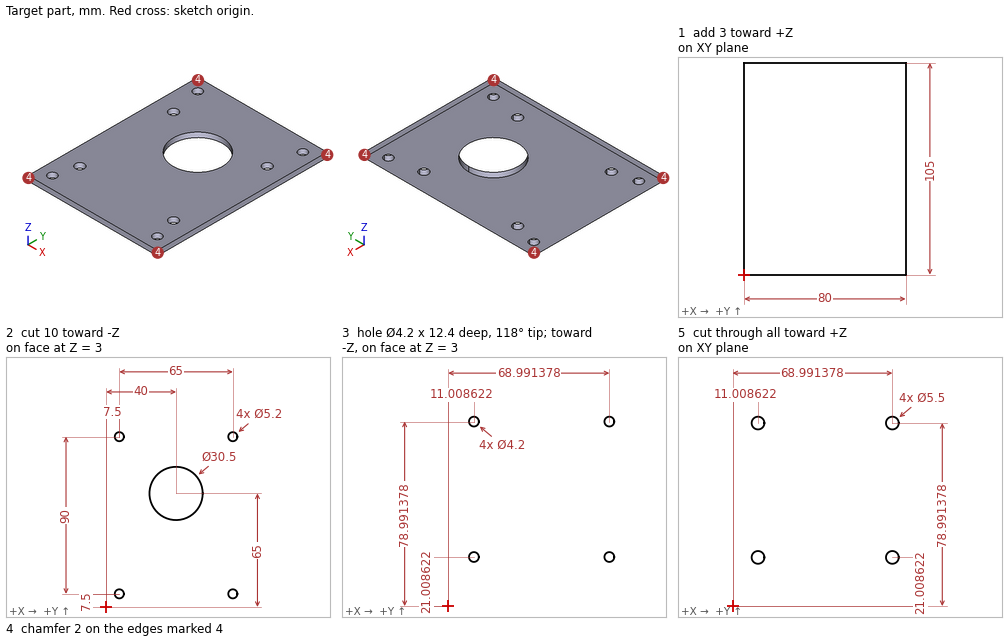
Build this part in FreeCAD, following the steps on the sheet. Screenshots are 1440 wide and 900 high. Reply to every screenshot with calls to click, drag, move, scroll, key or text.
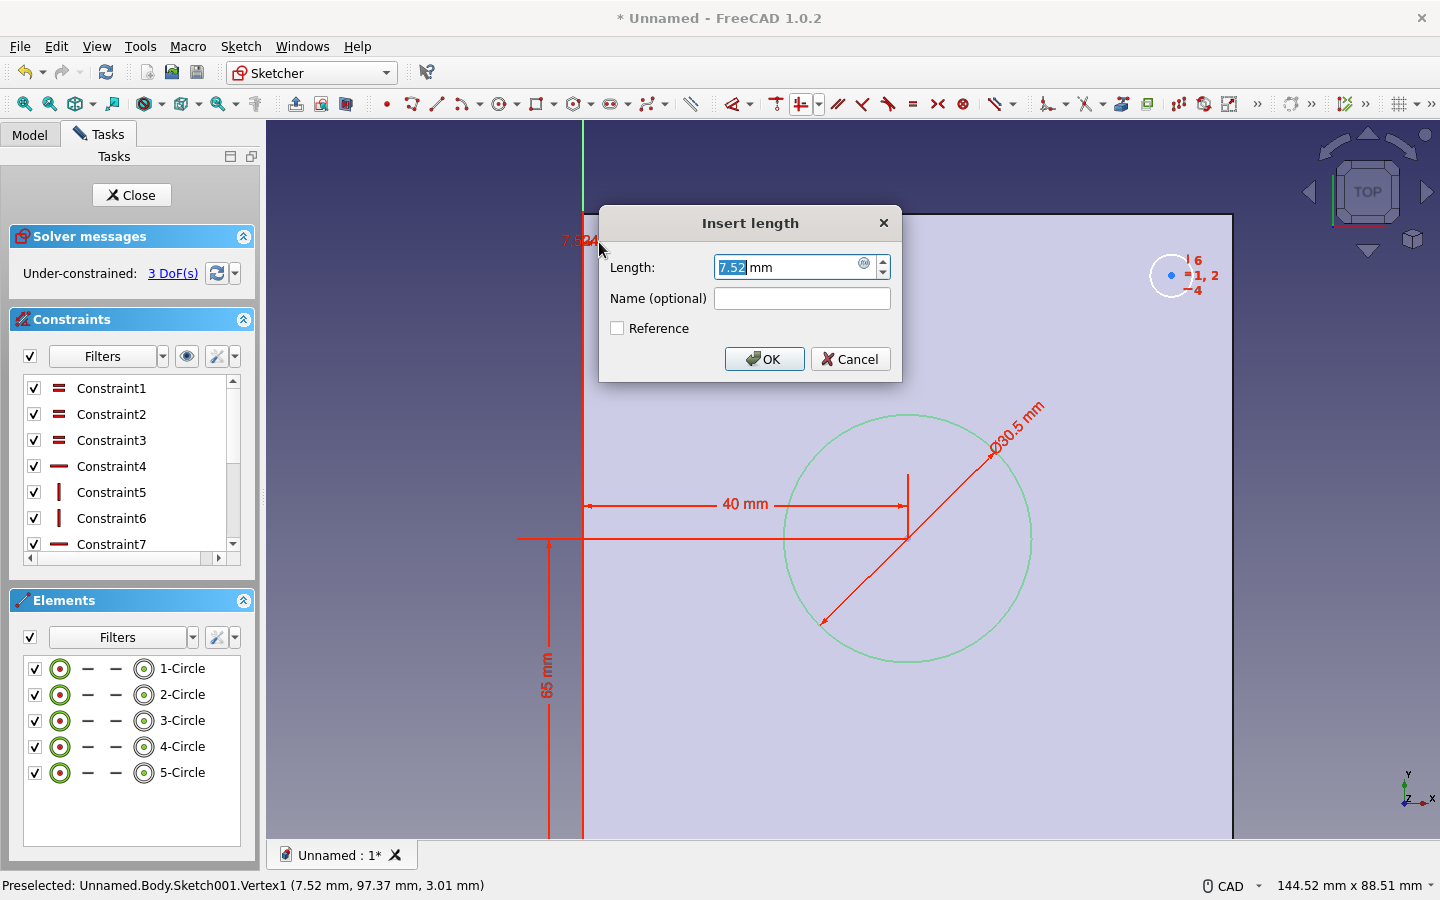
text(7.5)
key(Return)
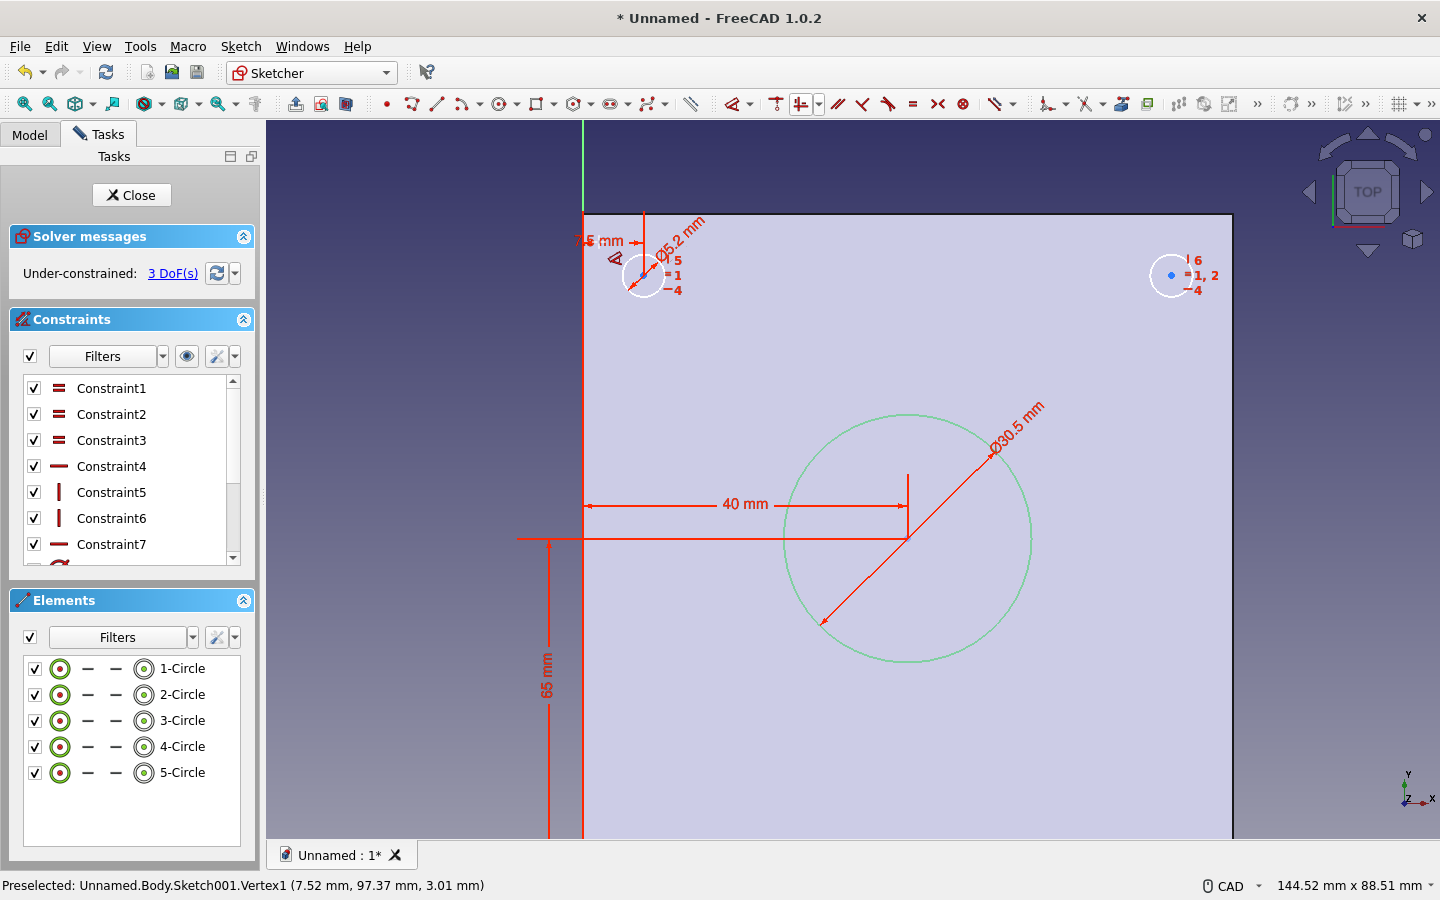
scroll(659, 260, down, 3)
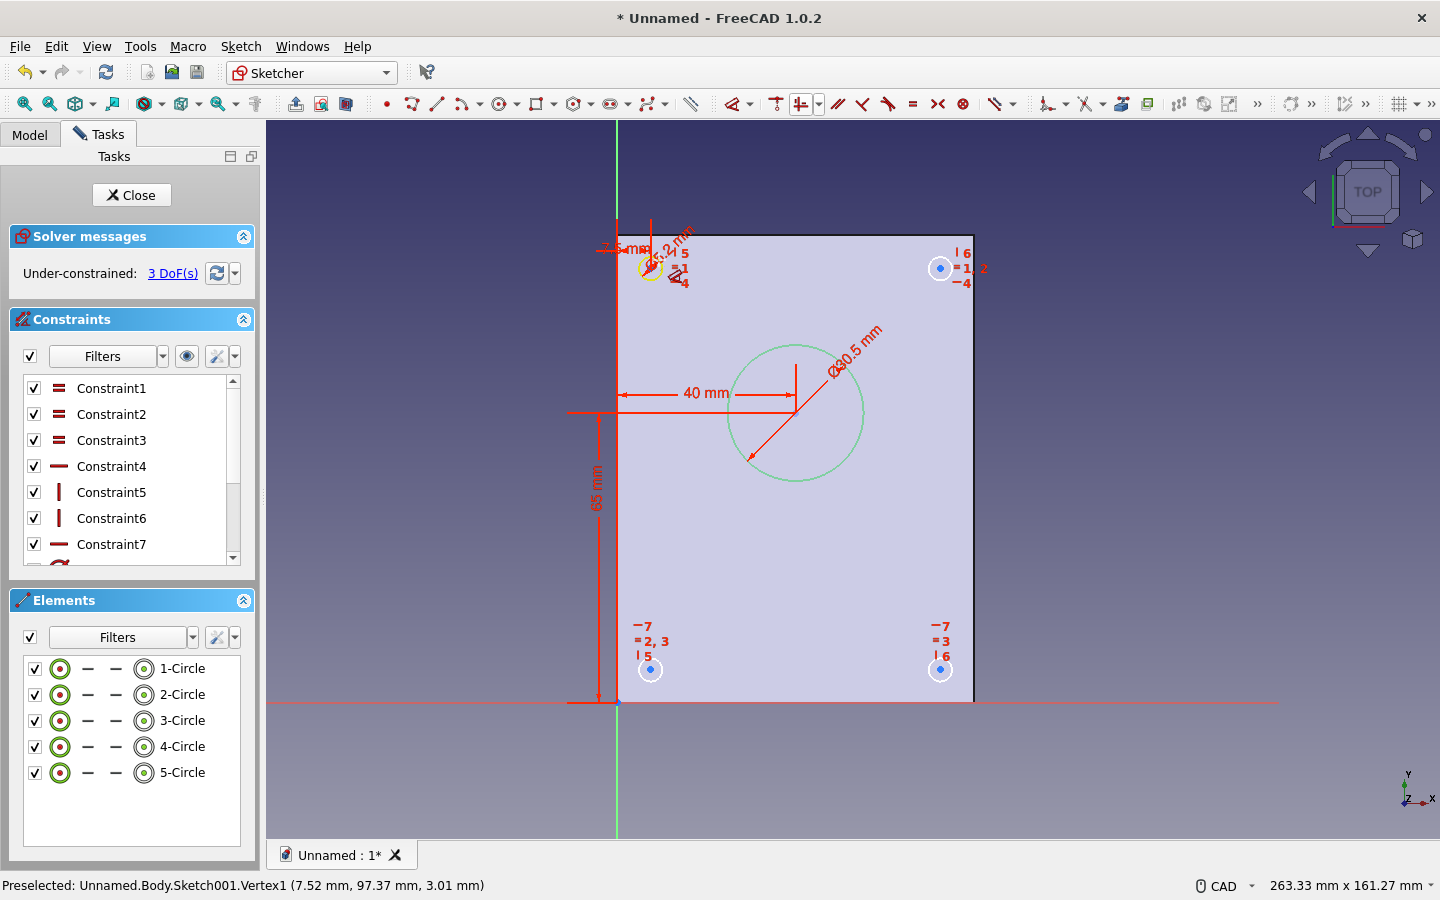
click(651, 670)
click(583, 686)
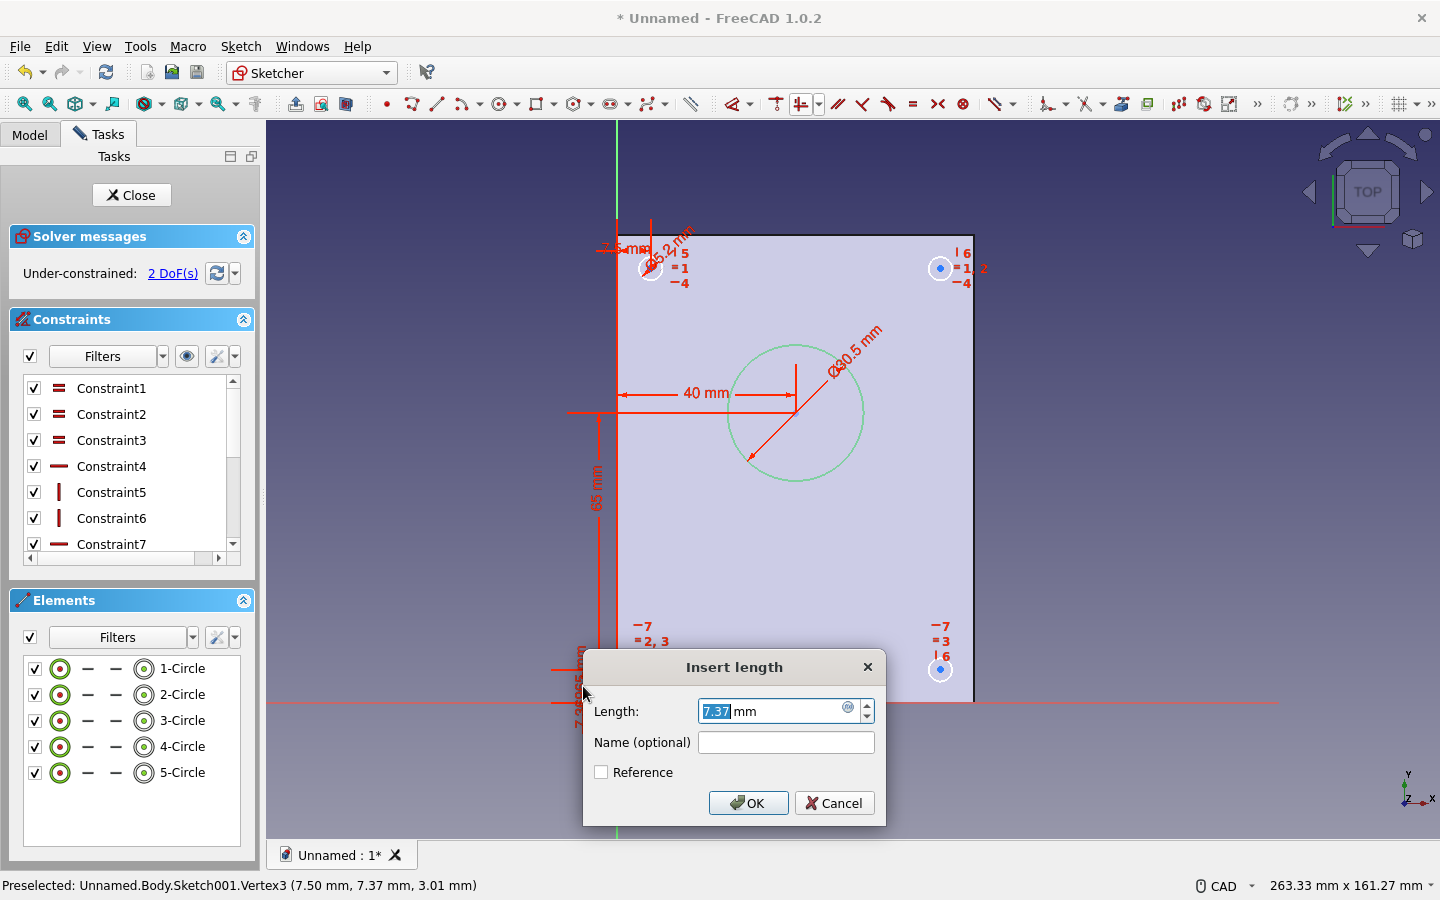
text(7.5)
key(Return)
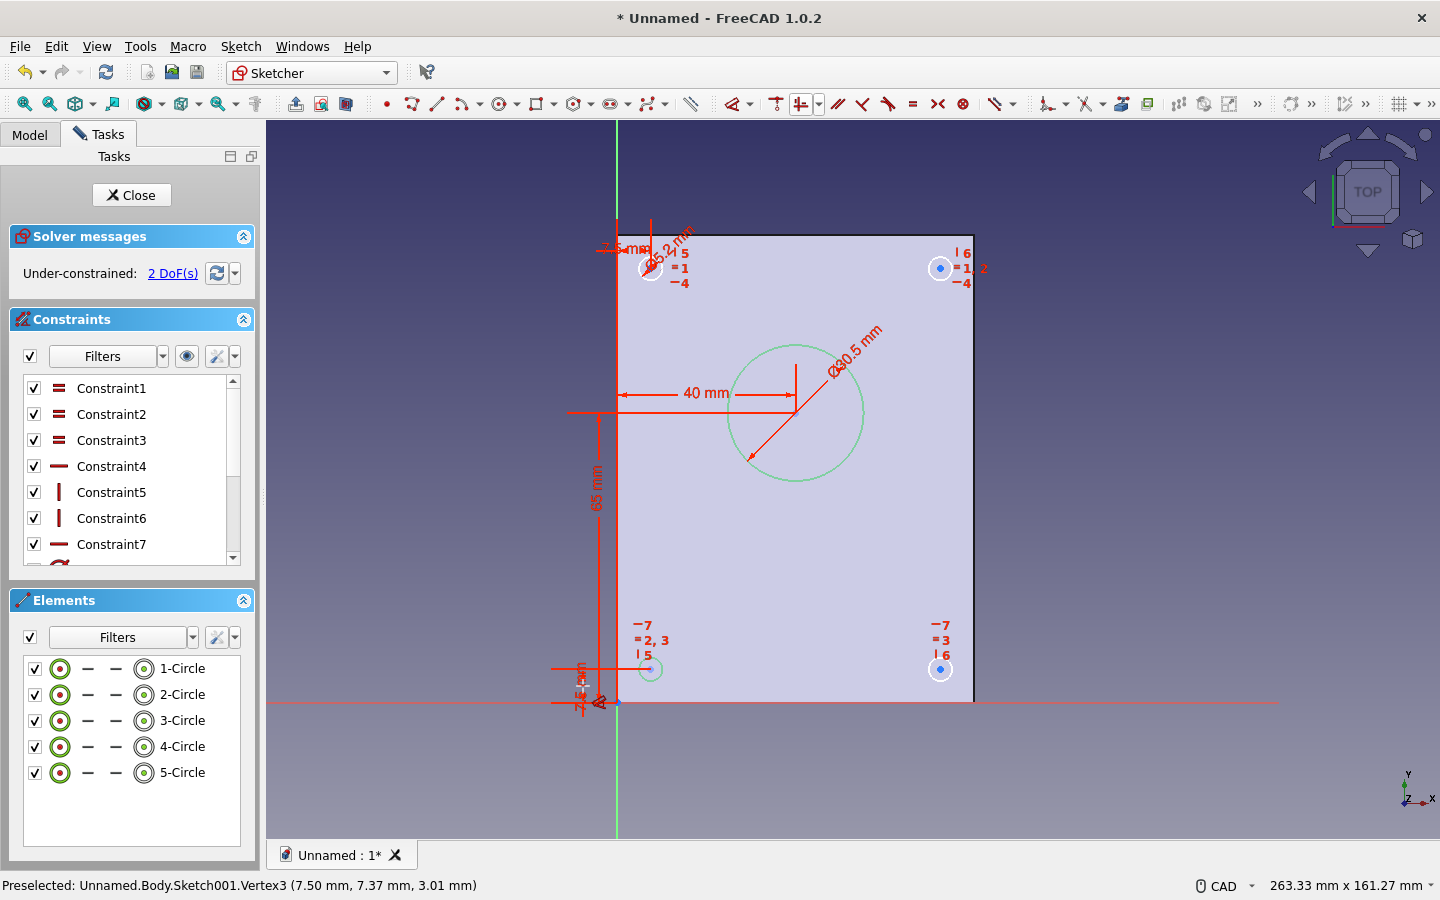
click(651, 269)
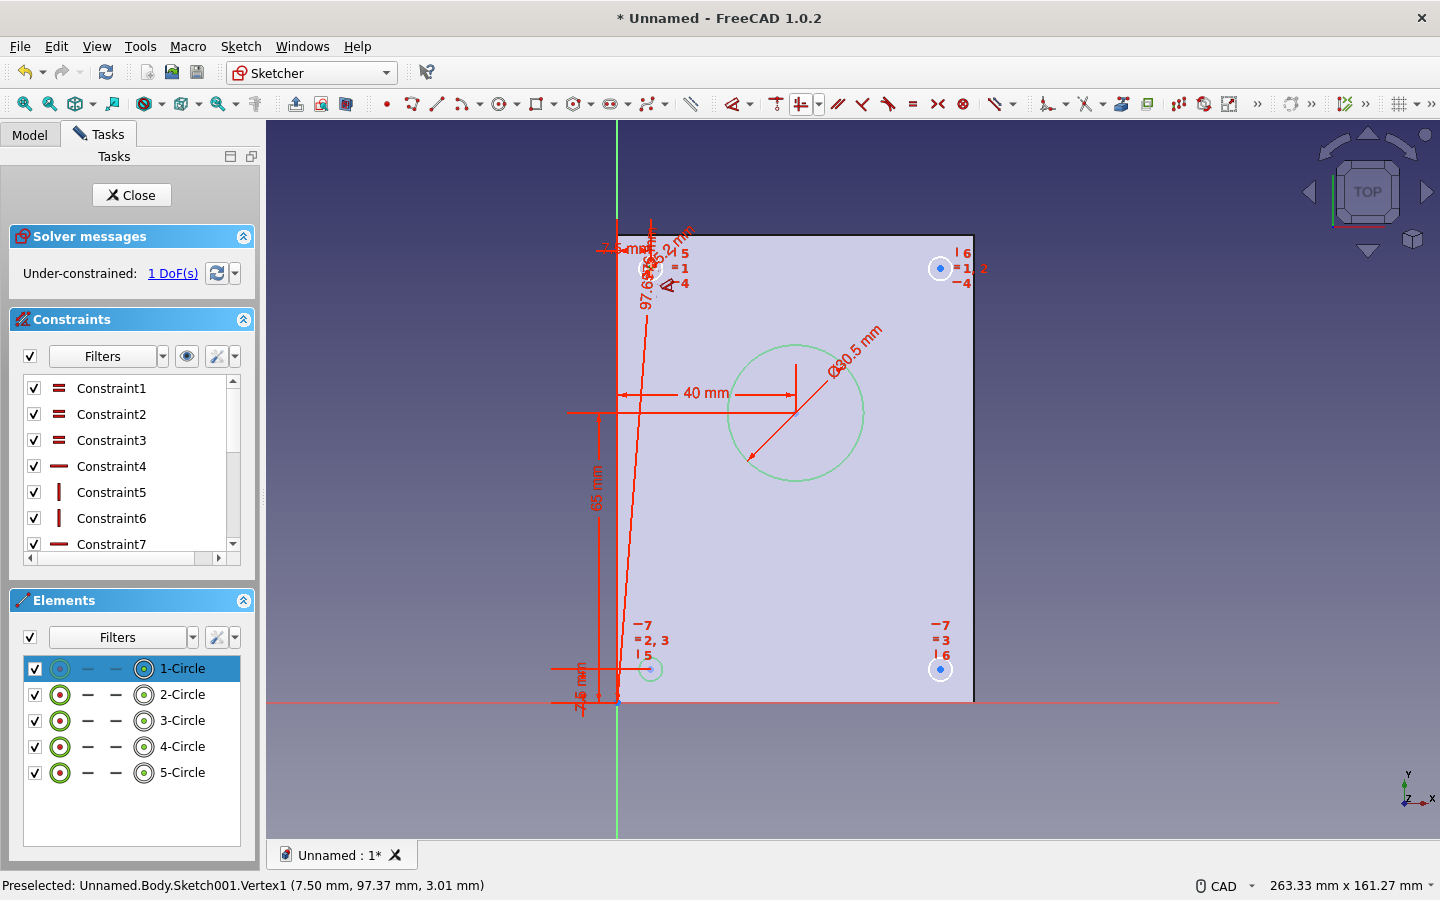
click(940, 269)
click(796, 235)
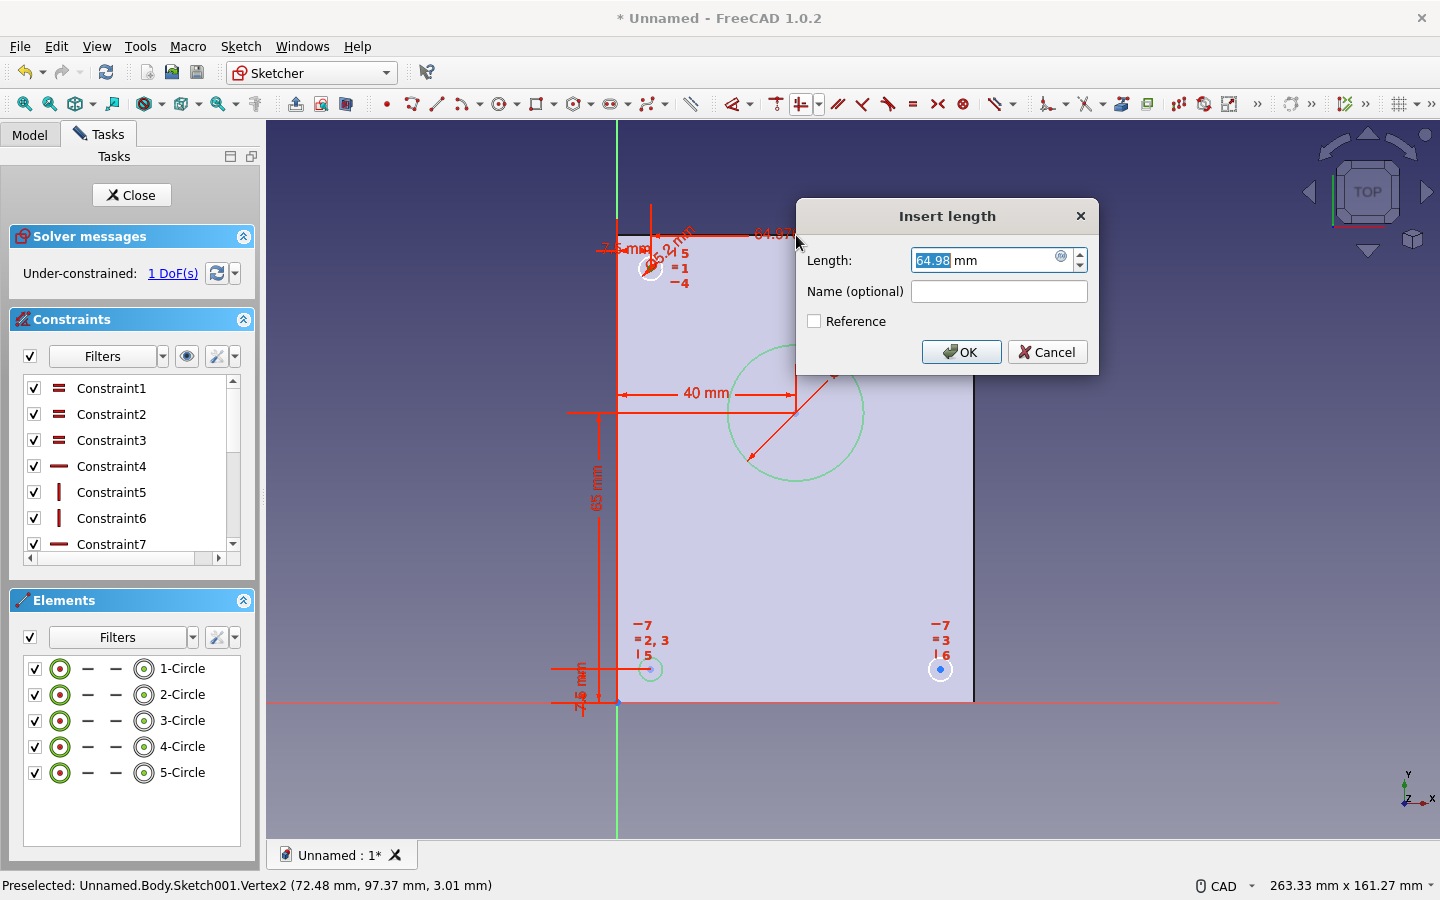
text(65)
key(Return)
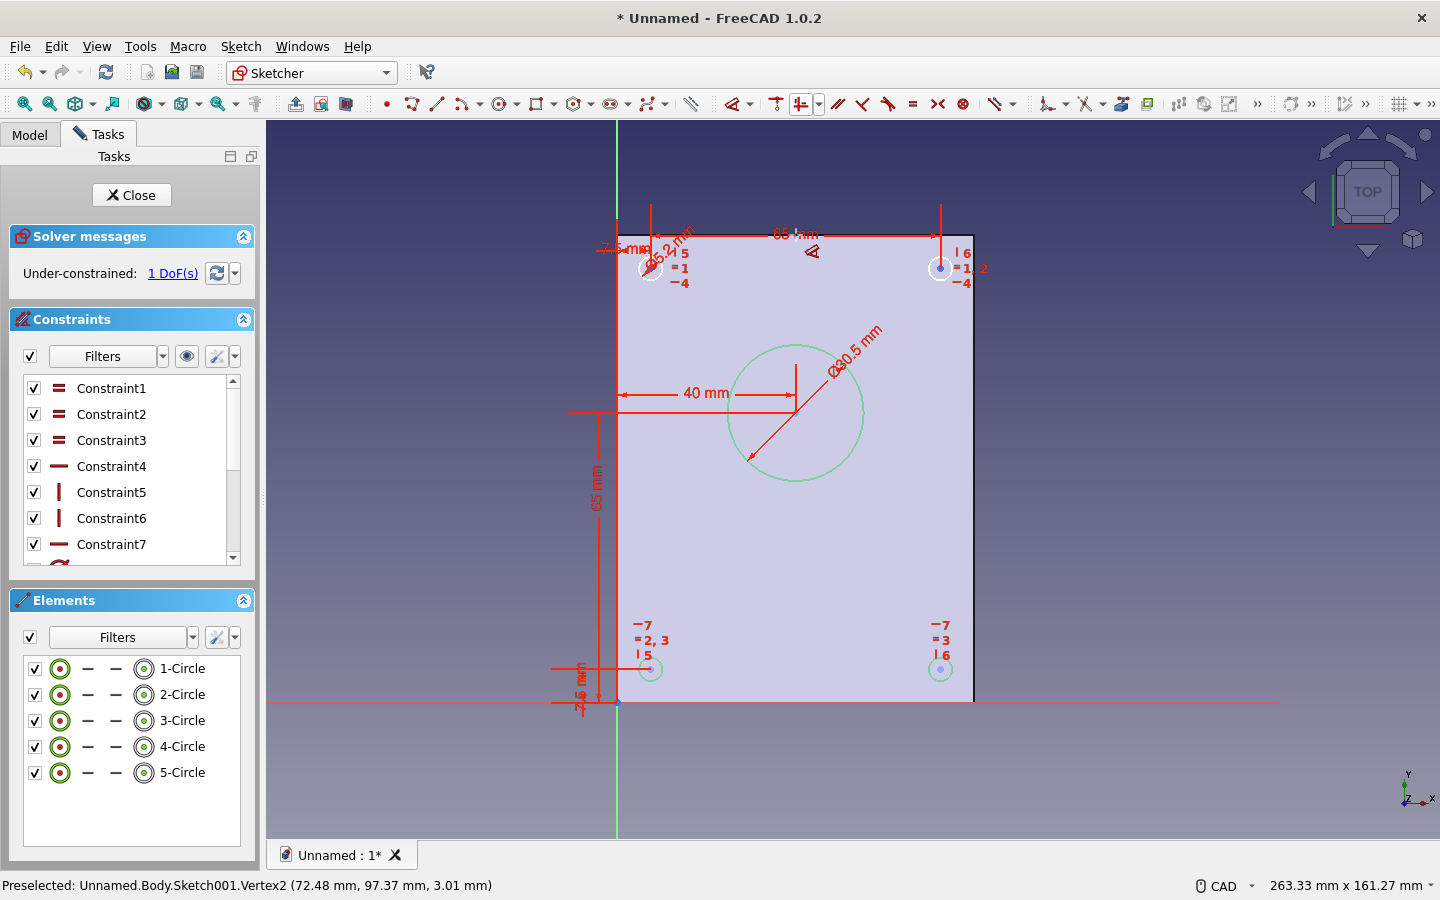
click(651, 269)